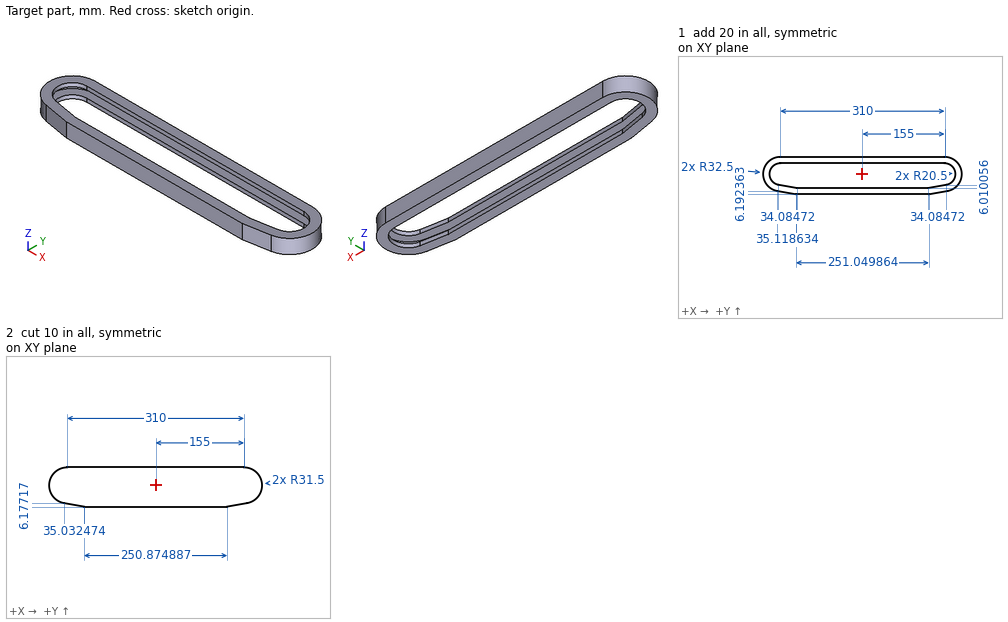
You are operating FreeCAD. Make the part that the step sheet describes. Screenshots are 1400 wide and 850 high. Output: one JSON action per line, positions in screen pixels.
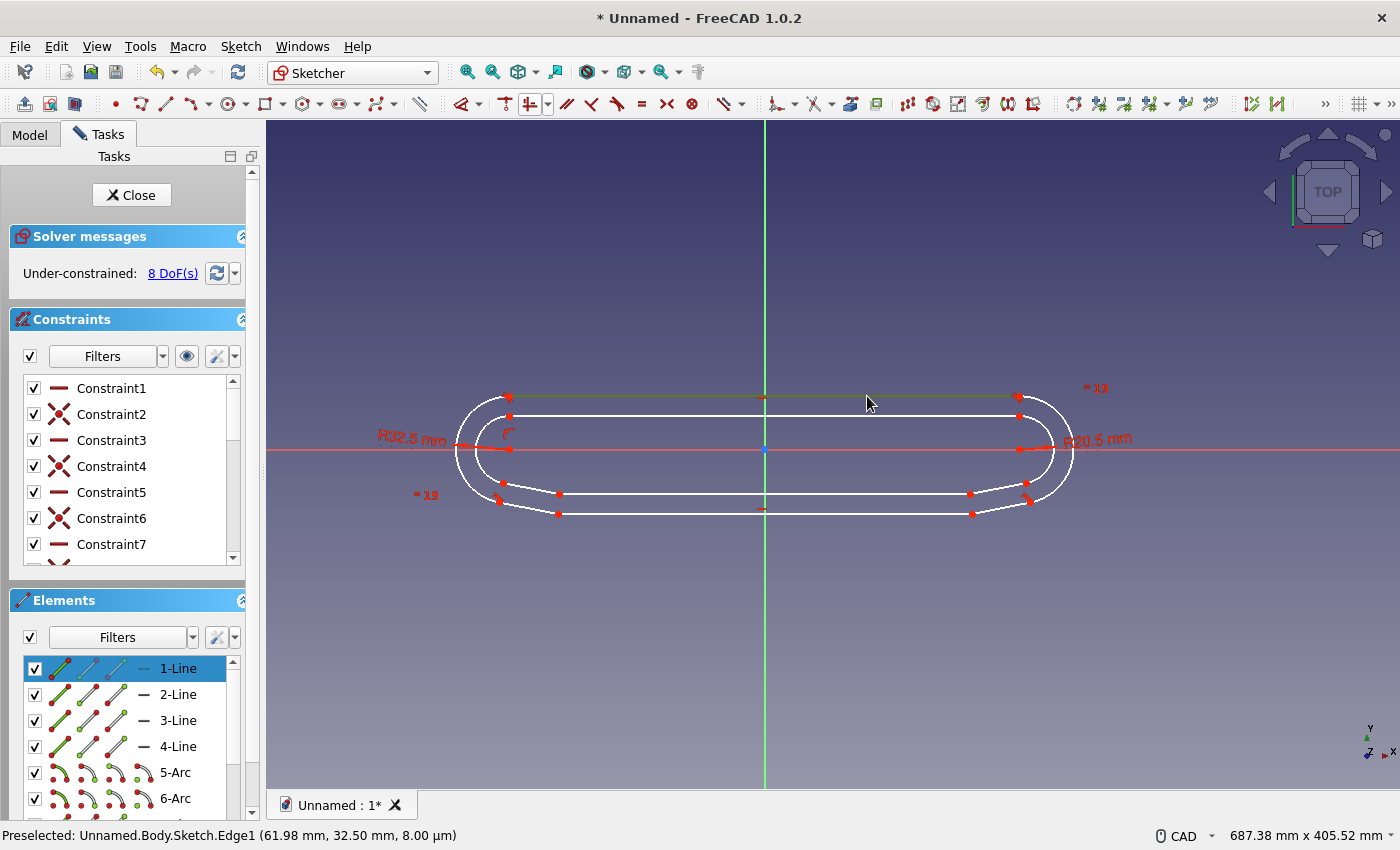
{"action": "key", "text": "l"}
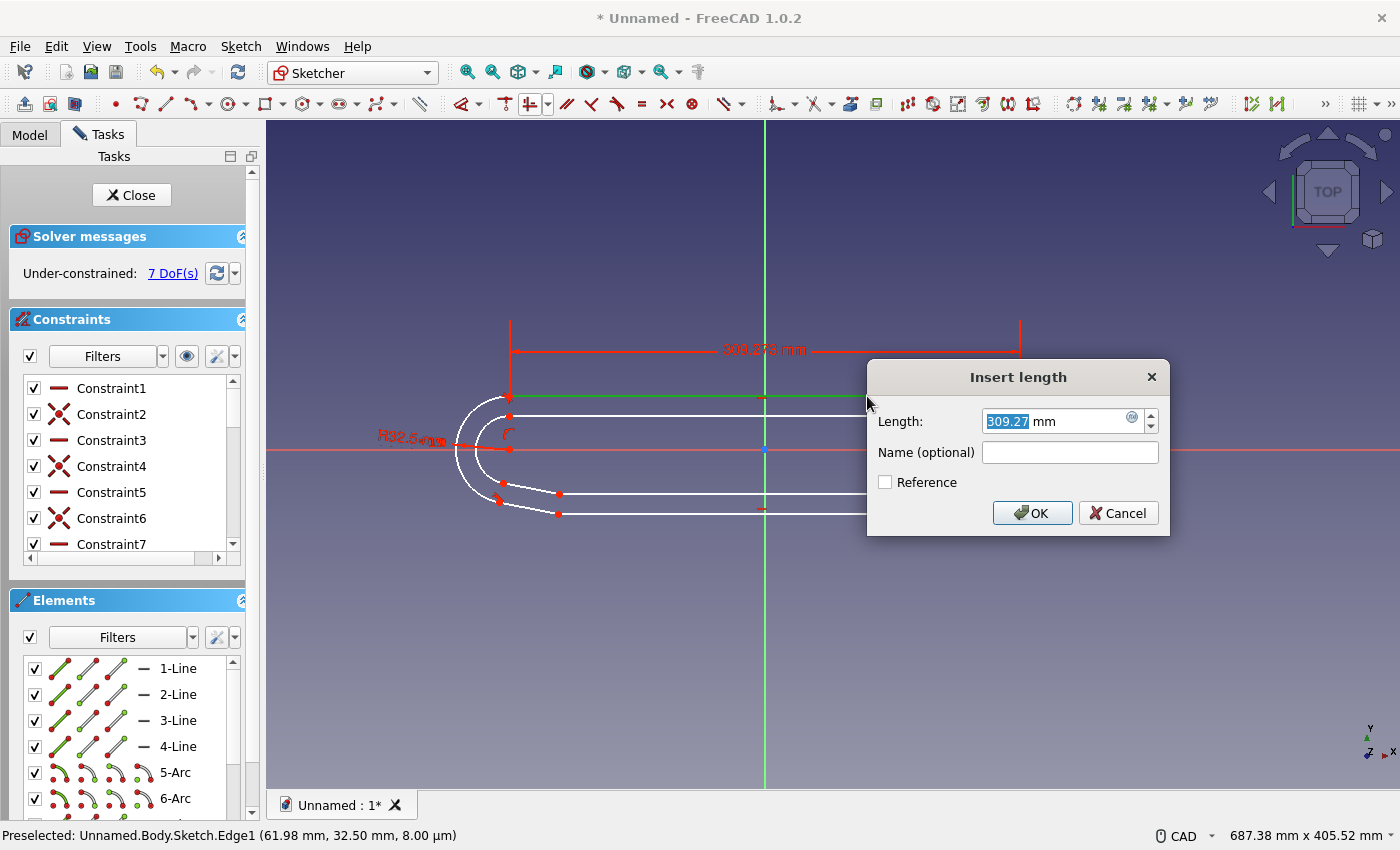
{"action": "type", "text": "310"}
{"action": "key", "text": "Return"}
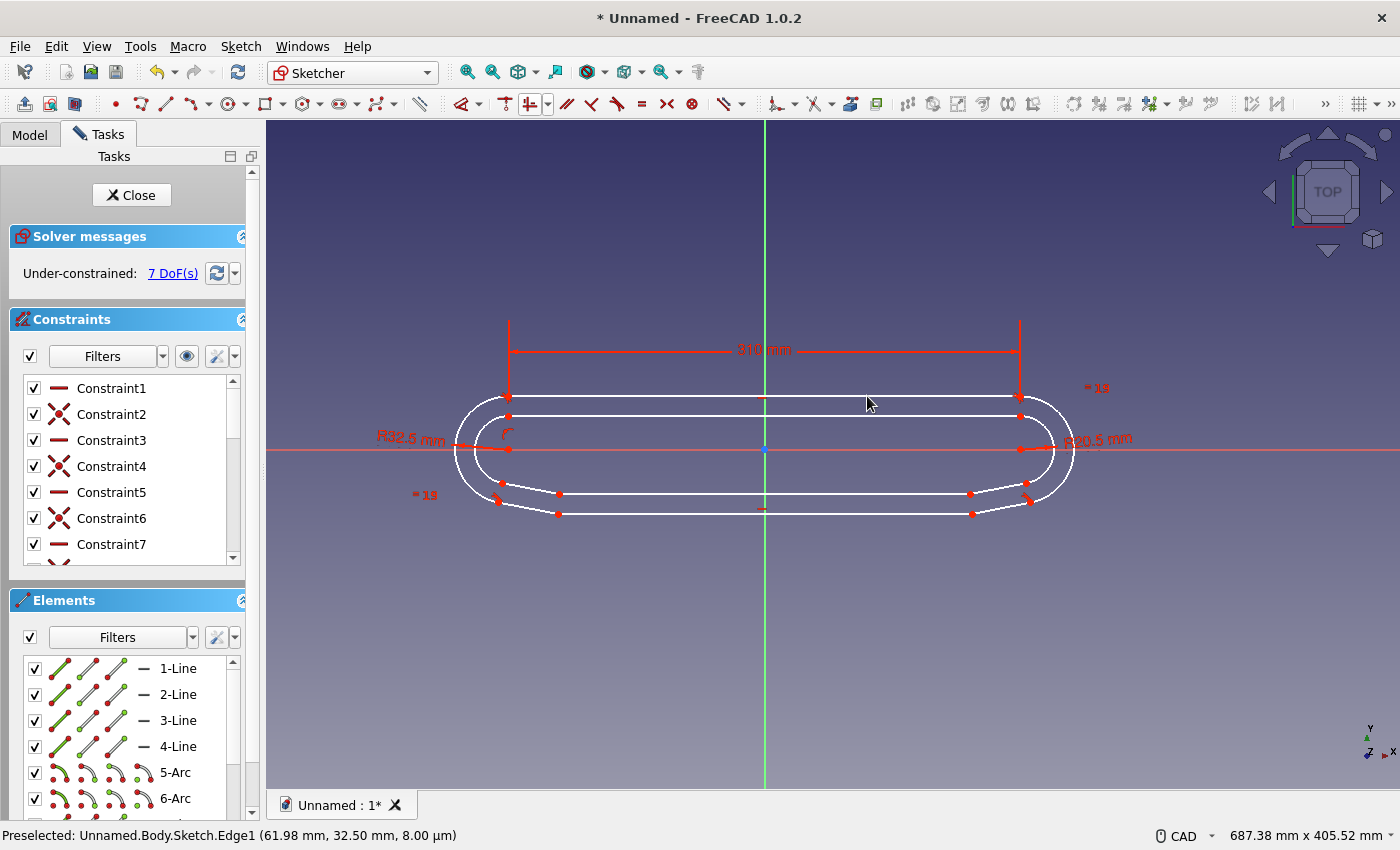
{"action": "left_click", "coordinate": [1020, 396]}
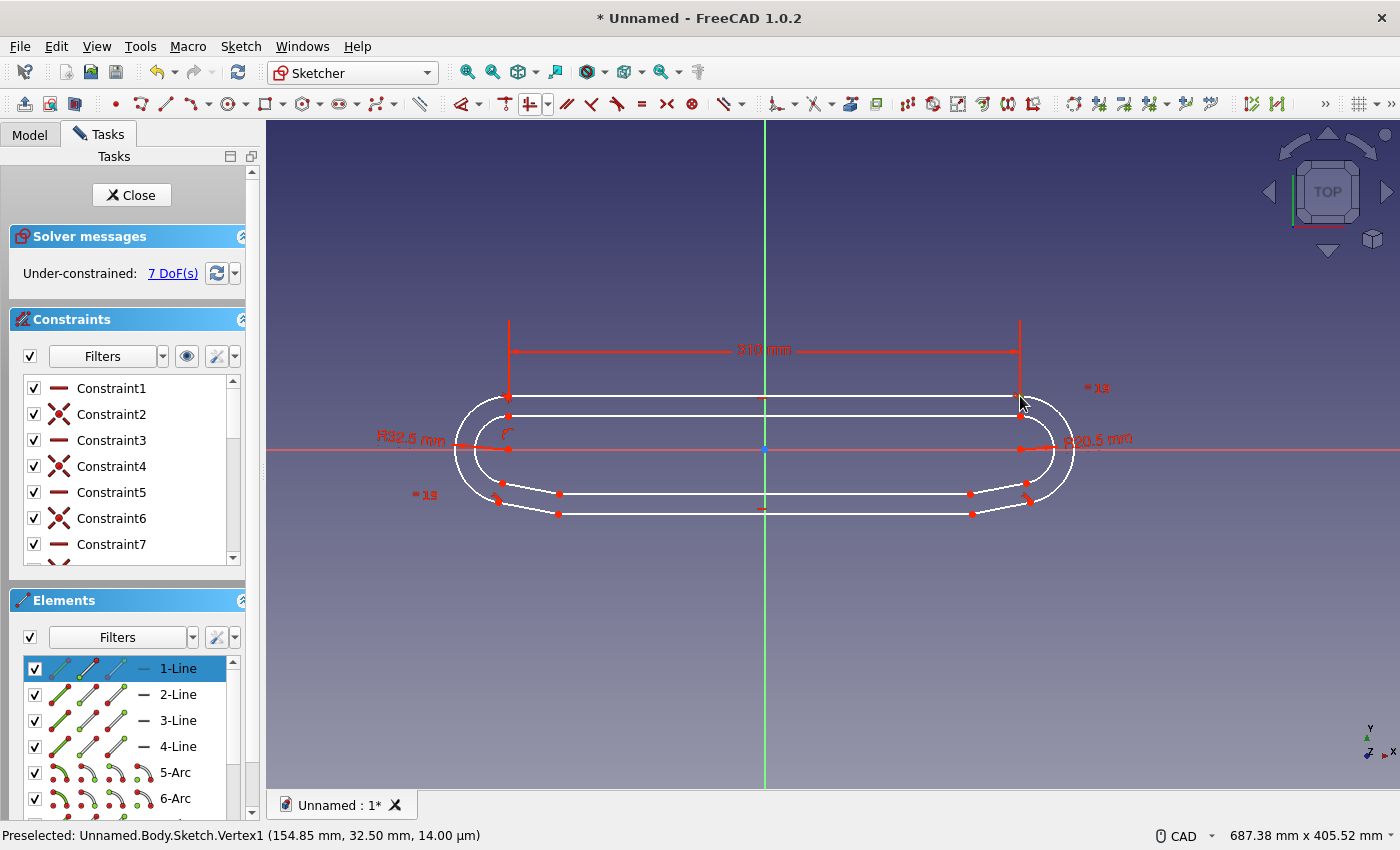
{"action": "key", "text": "l"}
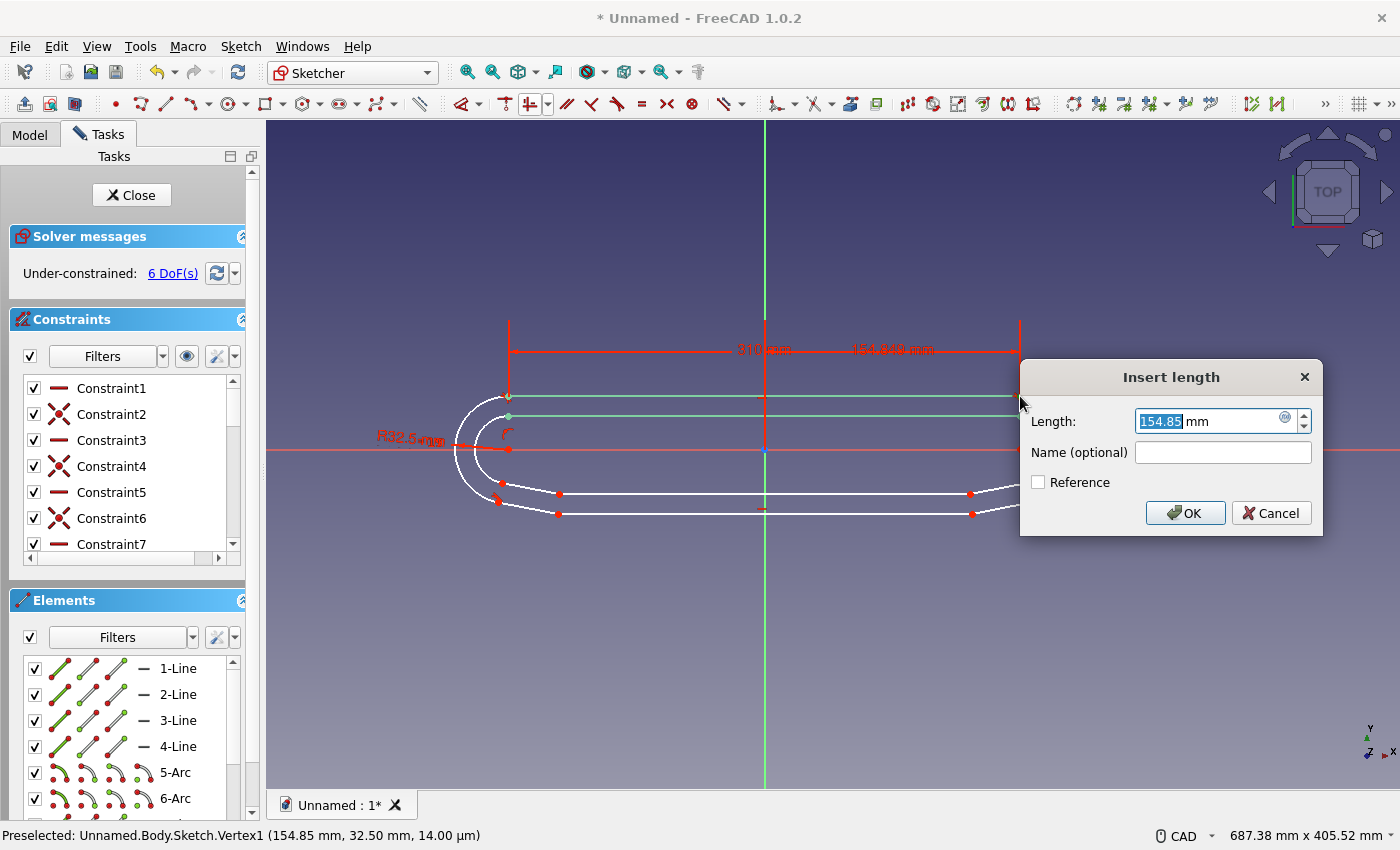
{"action": "type", "text": "155"}
{"action": "key", "text": "Return"}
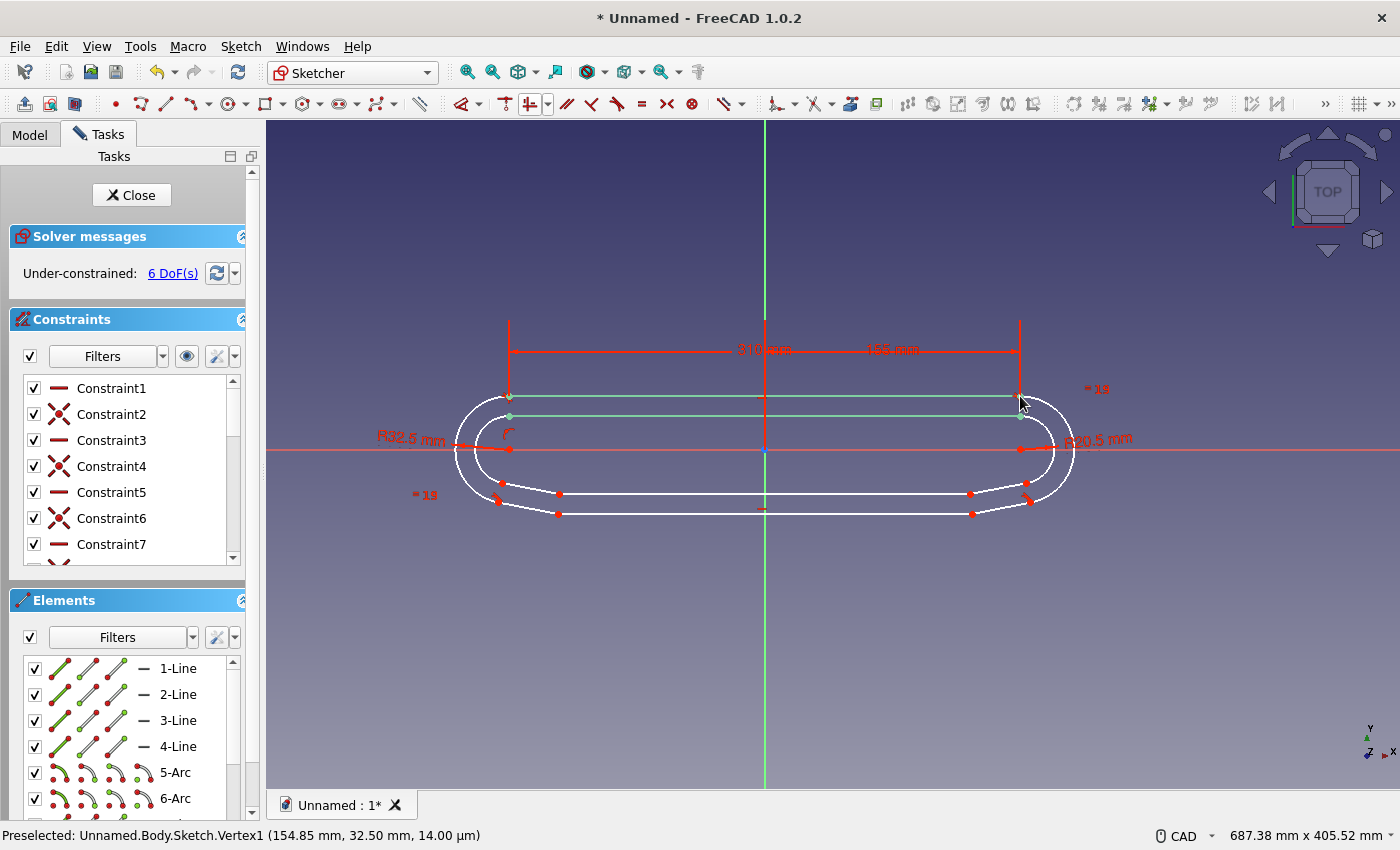
{"action": "scroll", "coordinate": [517, 506], "scroll_direction": "up", "scroll_amount": 7}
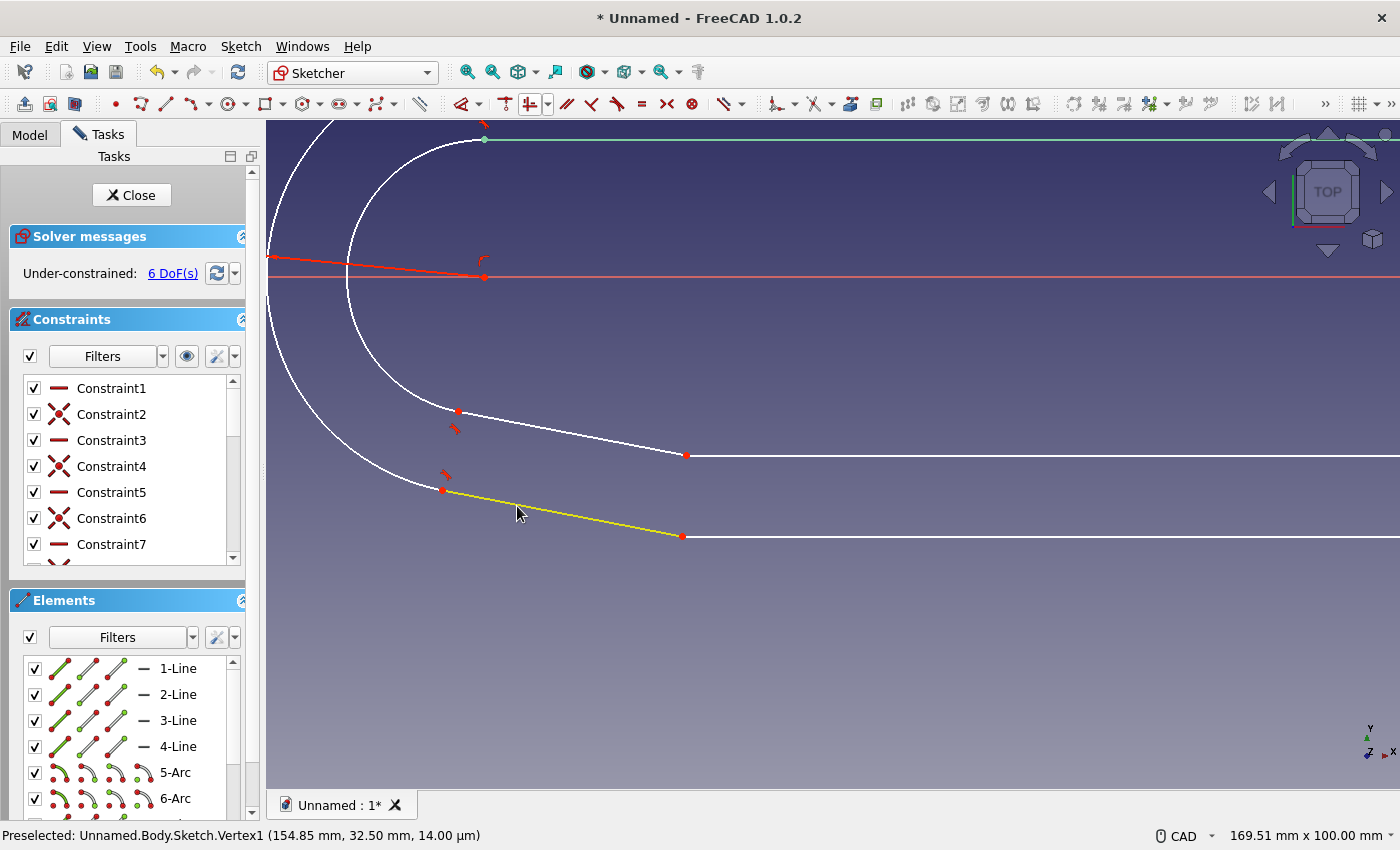
{"action": "left_click", "coordinate": [515, 504]}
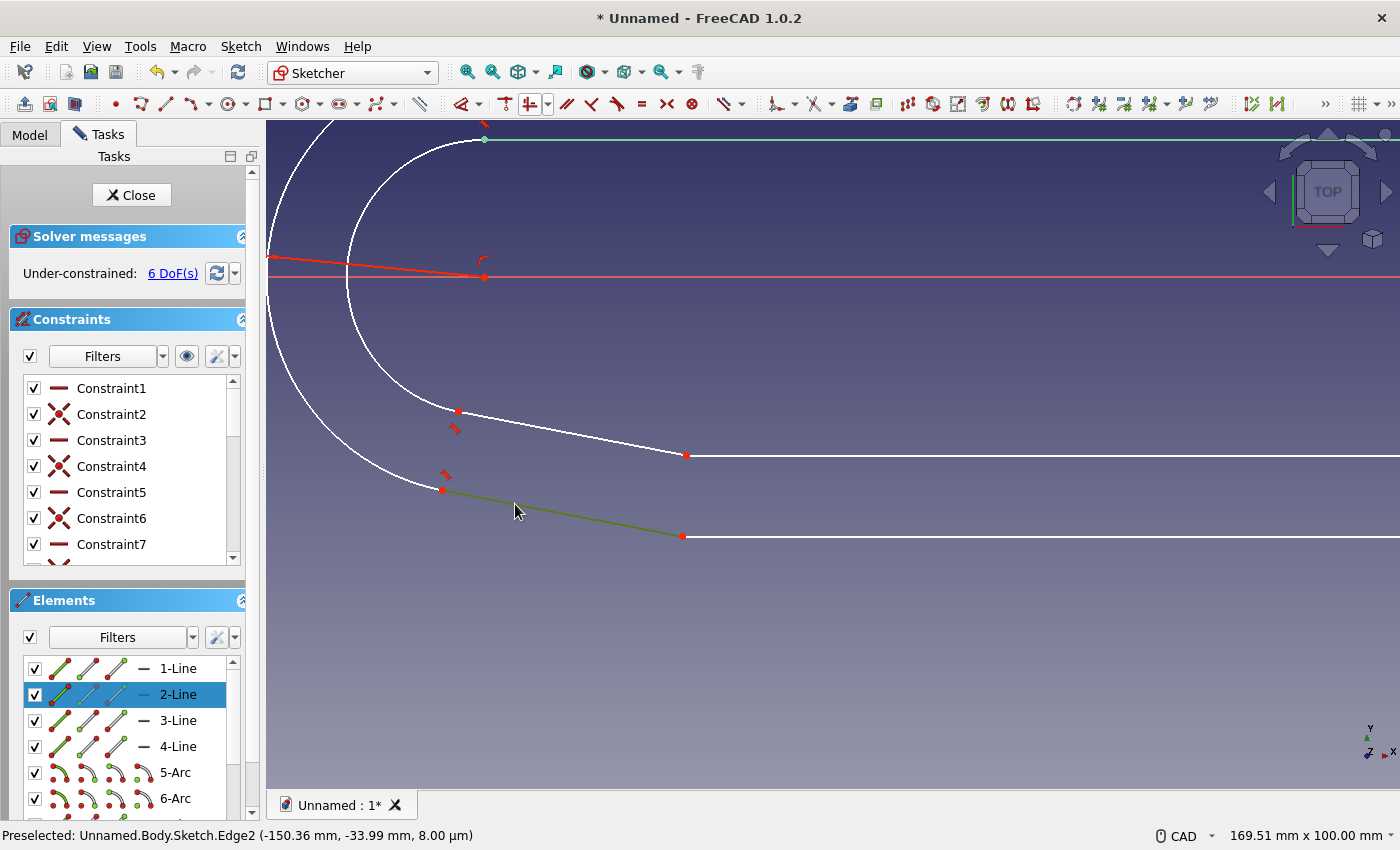
{"action": "key", "text": "i"}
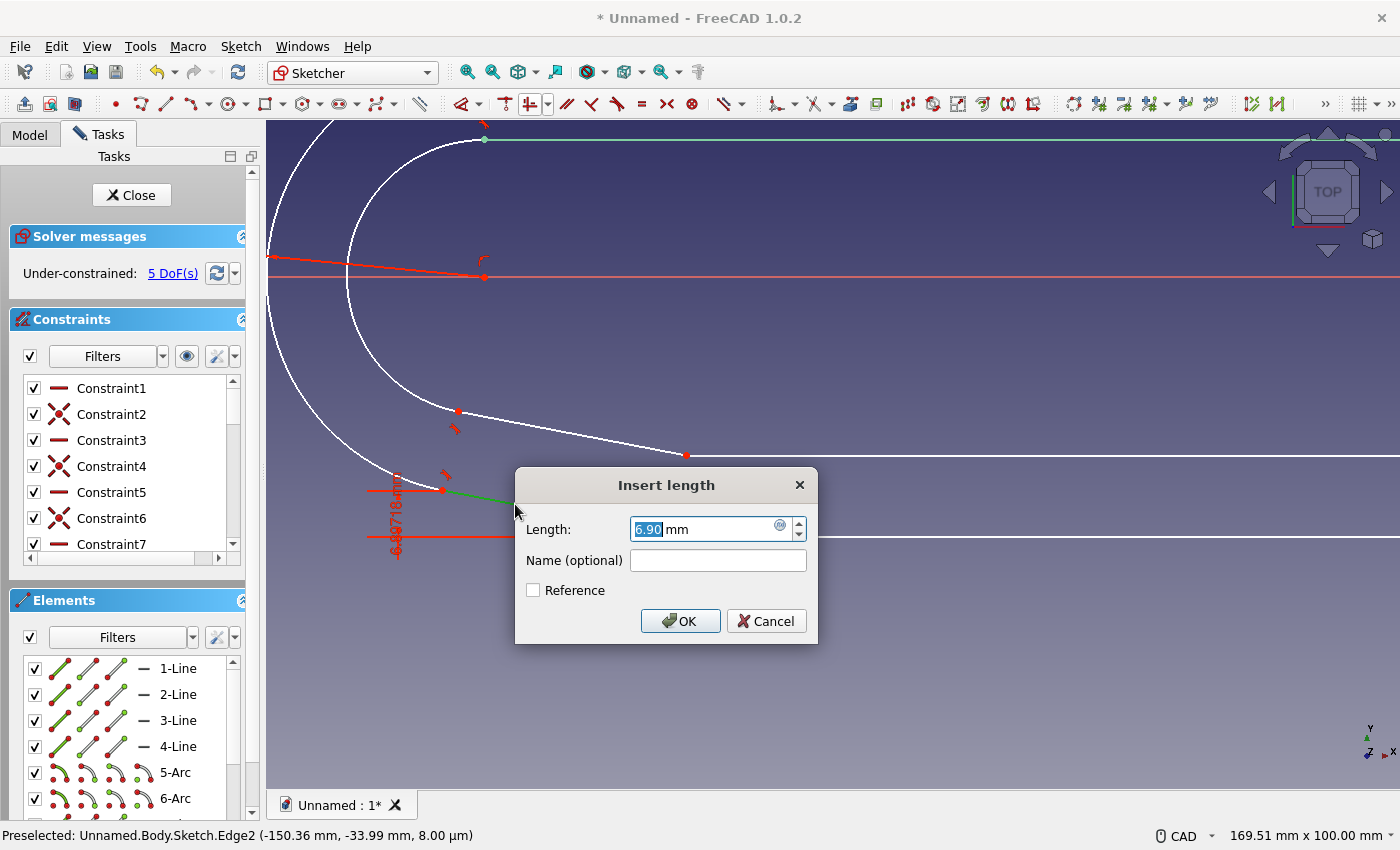
{"action": "type", "text": "6.192363"}
{"action": "key", "text": "Return"}